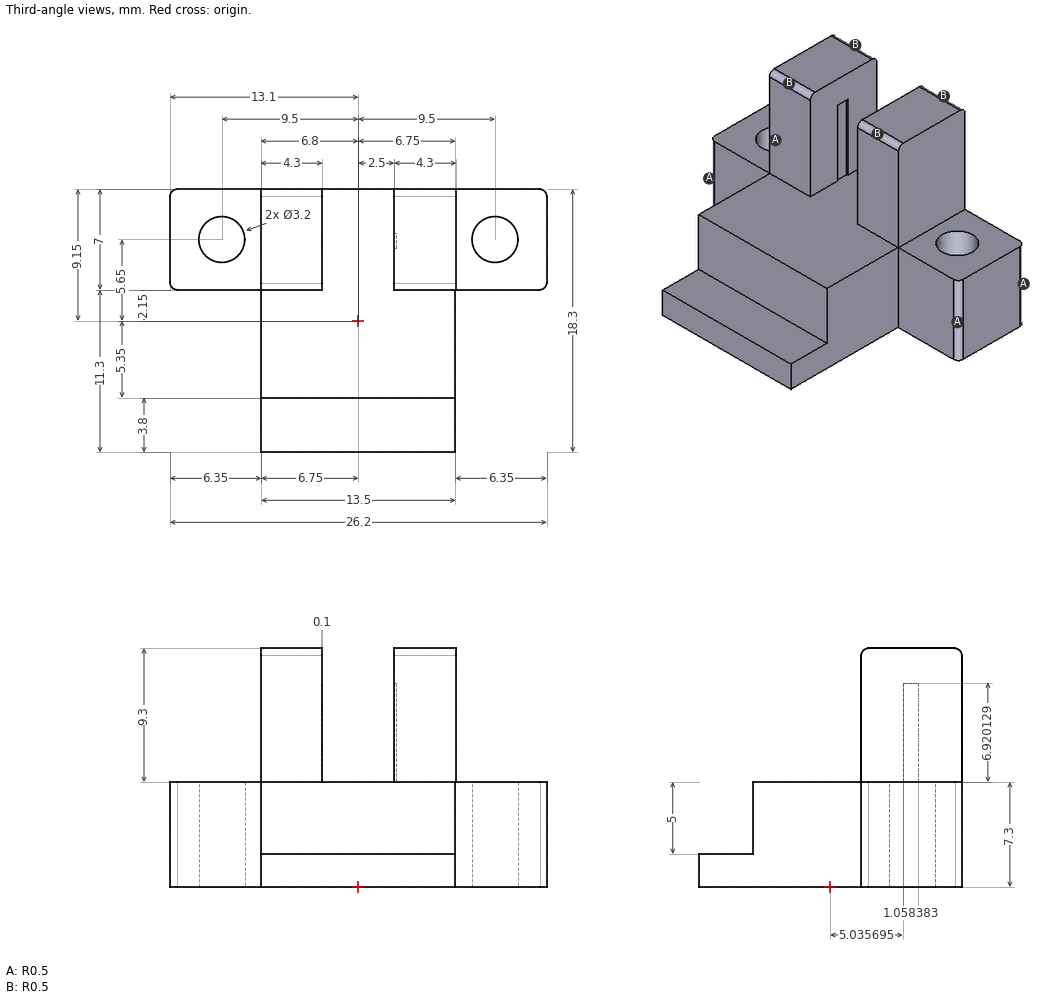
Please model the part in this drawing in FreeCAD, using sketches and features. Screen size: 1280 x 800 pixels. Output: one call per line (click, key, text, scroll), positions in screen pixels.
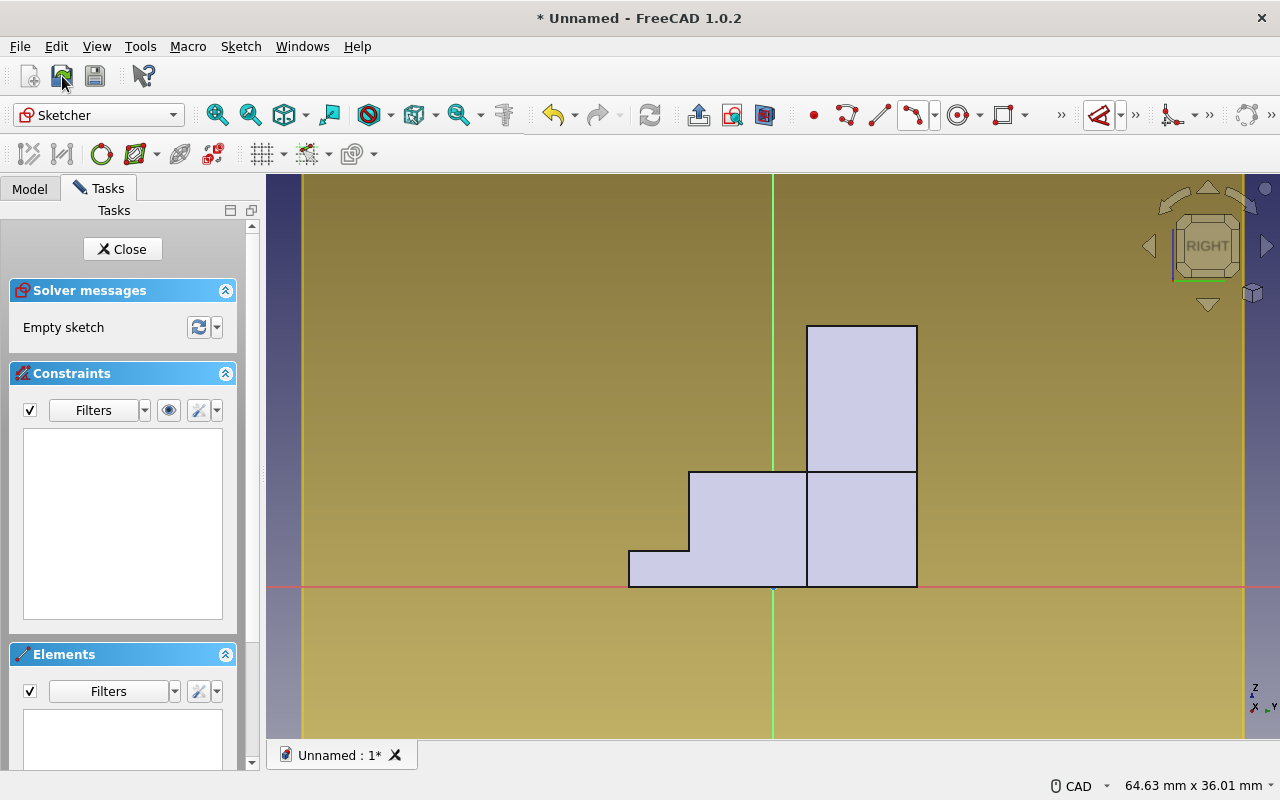
key(q)
key(s)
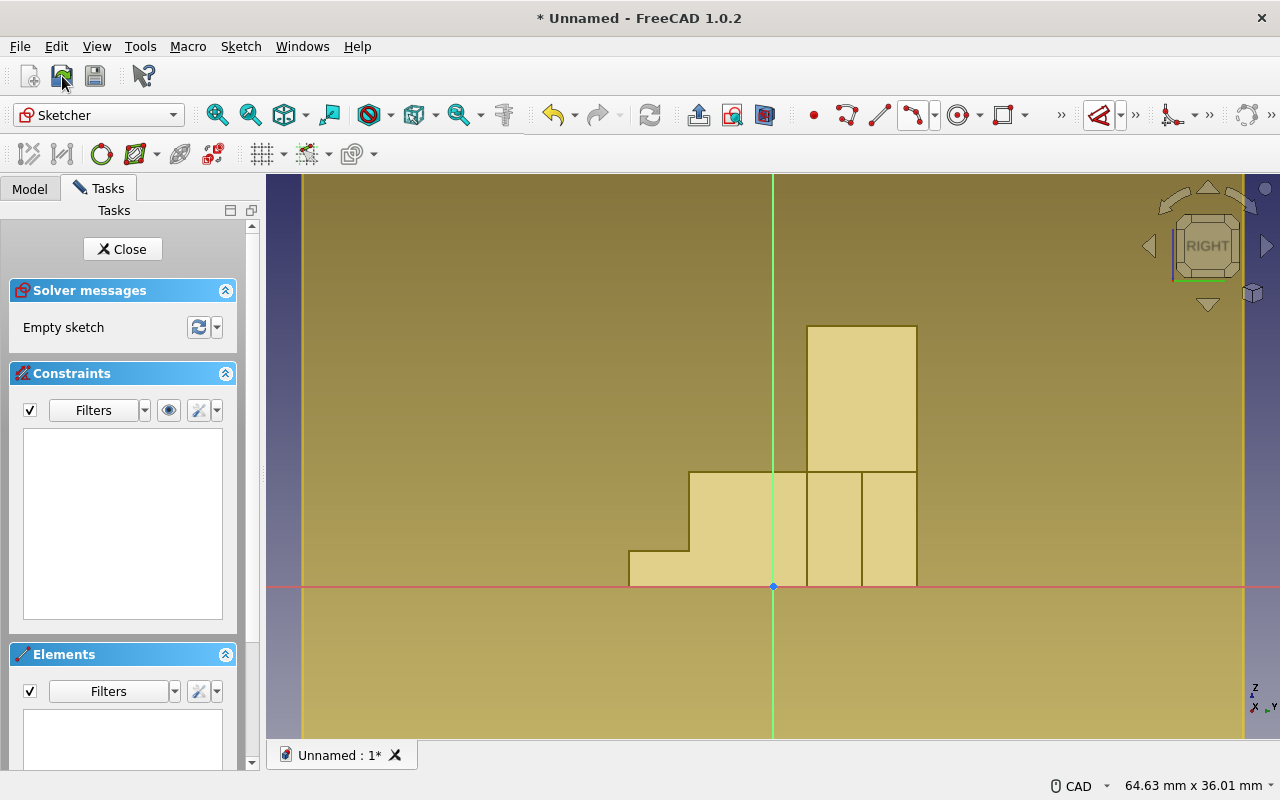
scroll(1057, 513, up, 2)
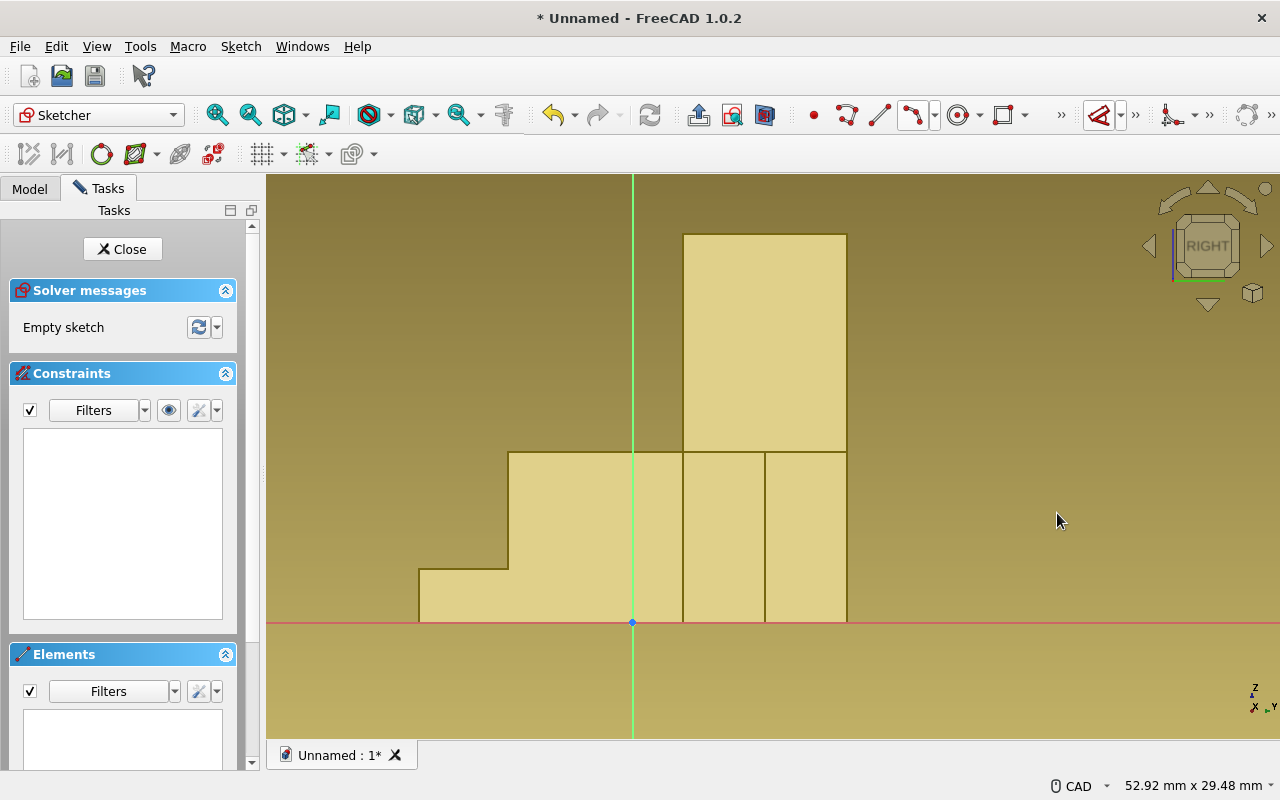
key(g)
key(r)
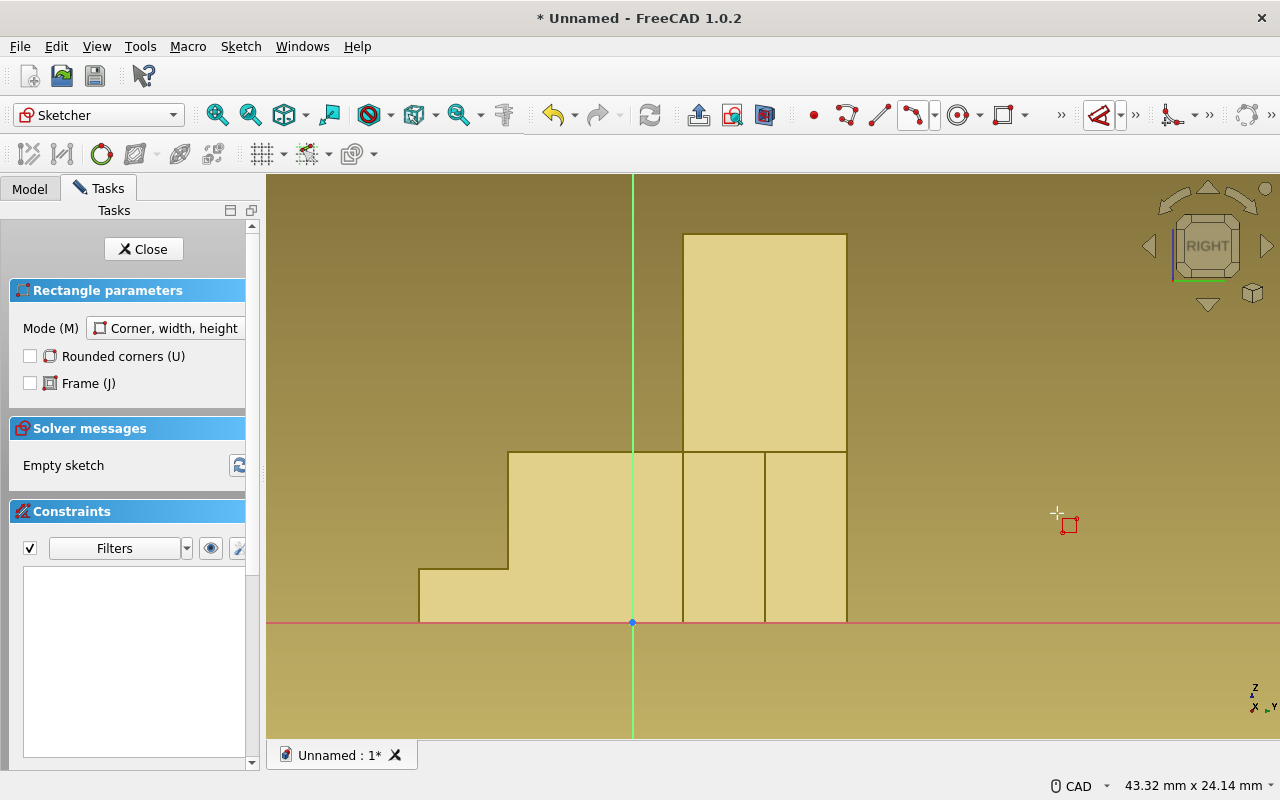
click(751, 290)
click(776, 452)
key(Escape)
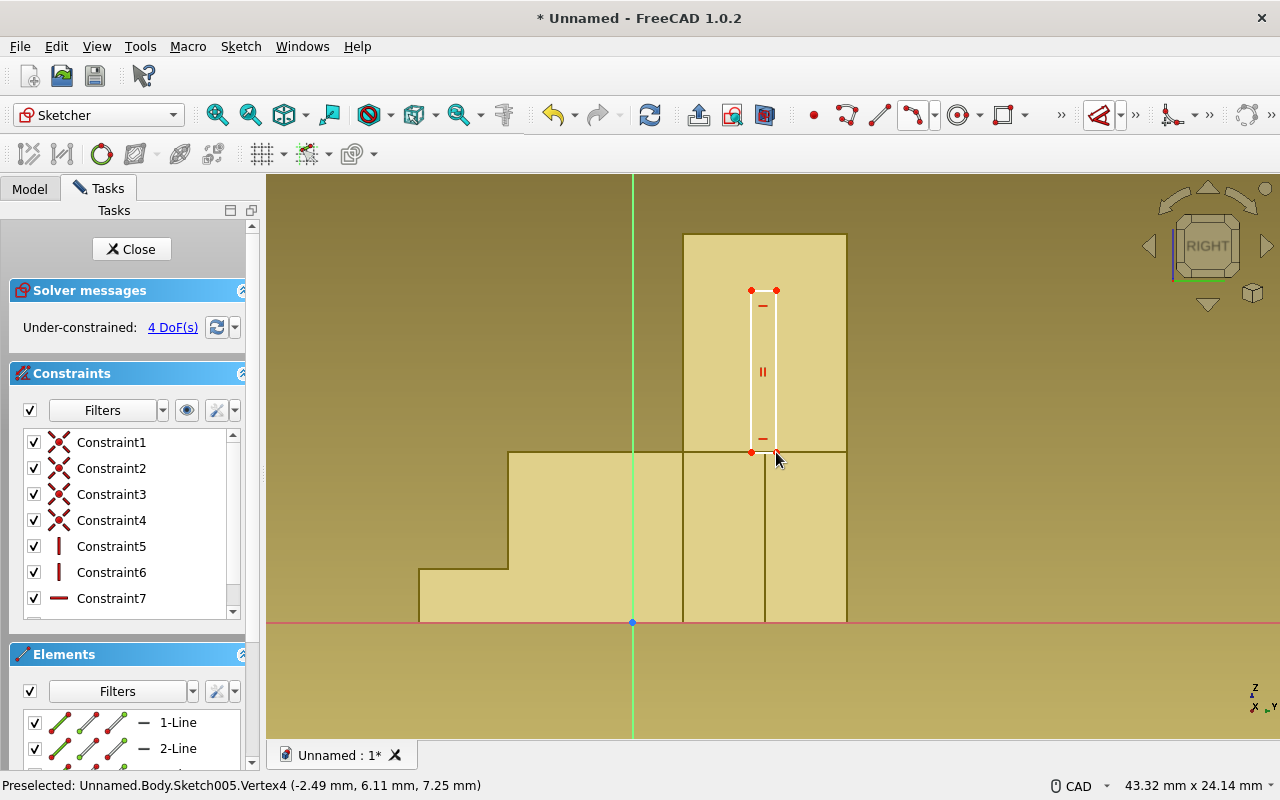
click(751, 453)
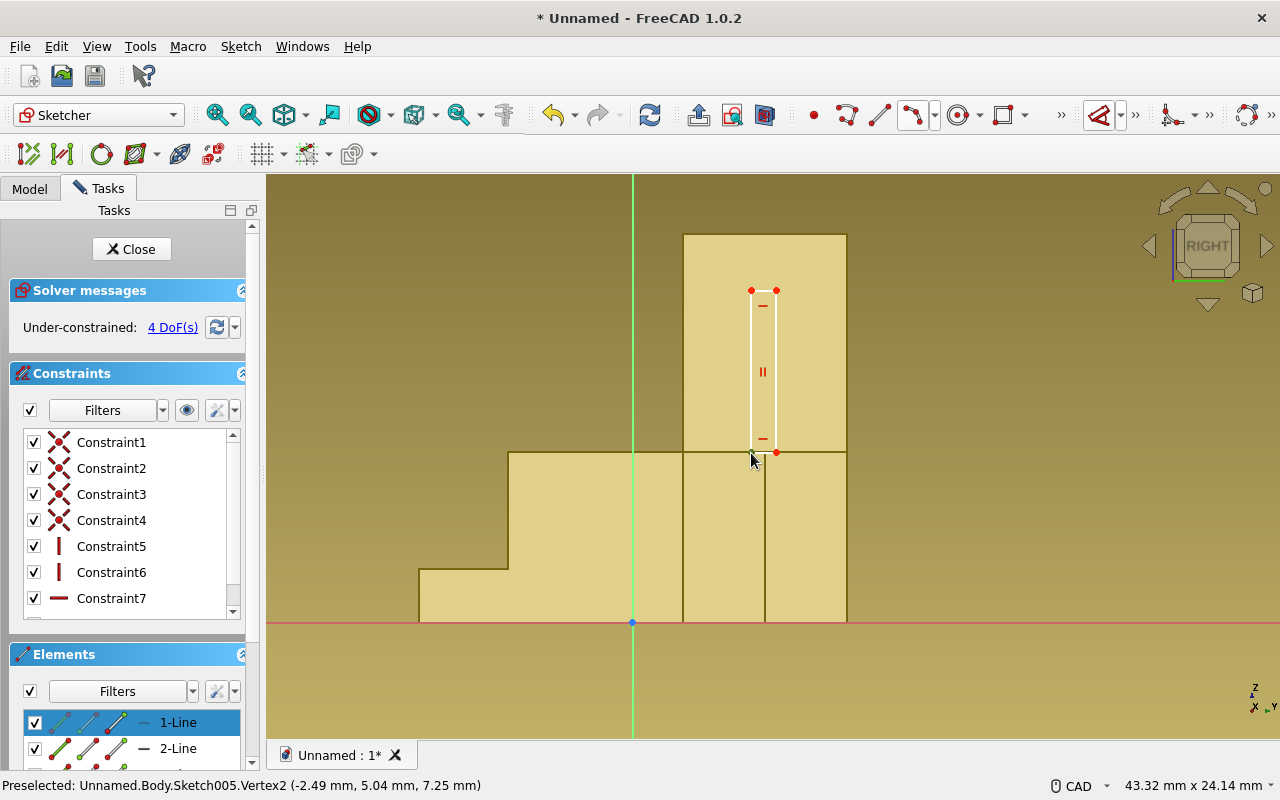
key(i)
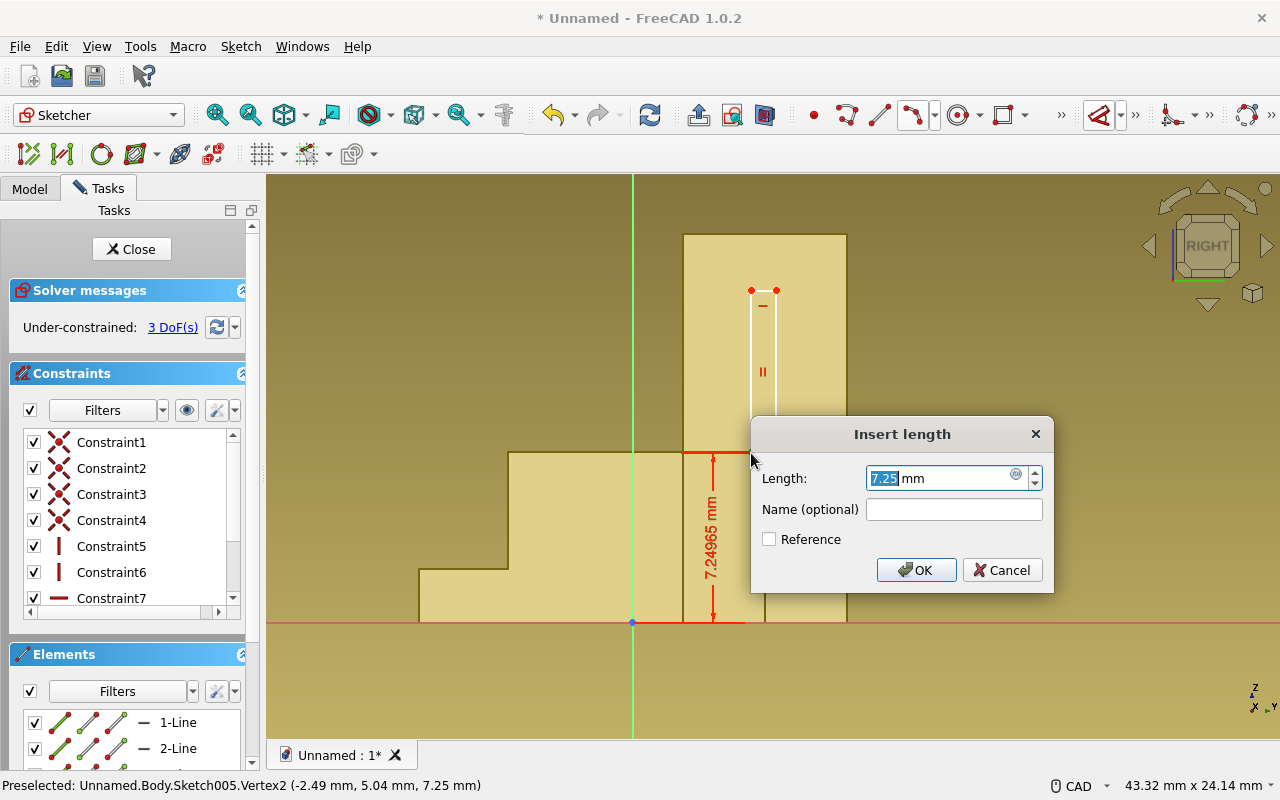
text(7.3)
key(Return)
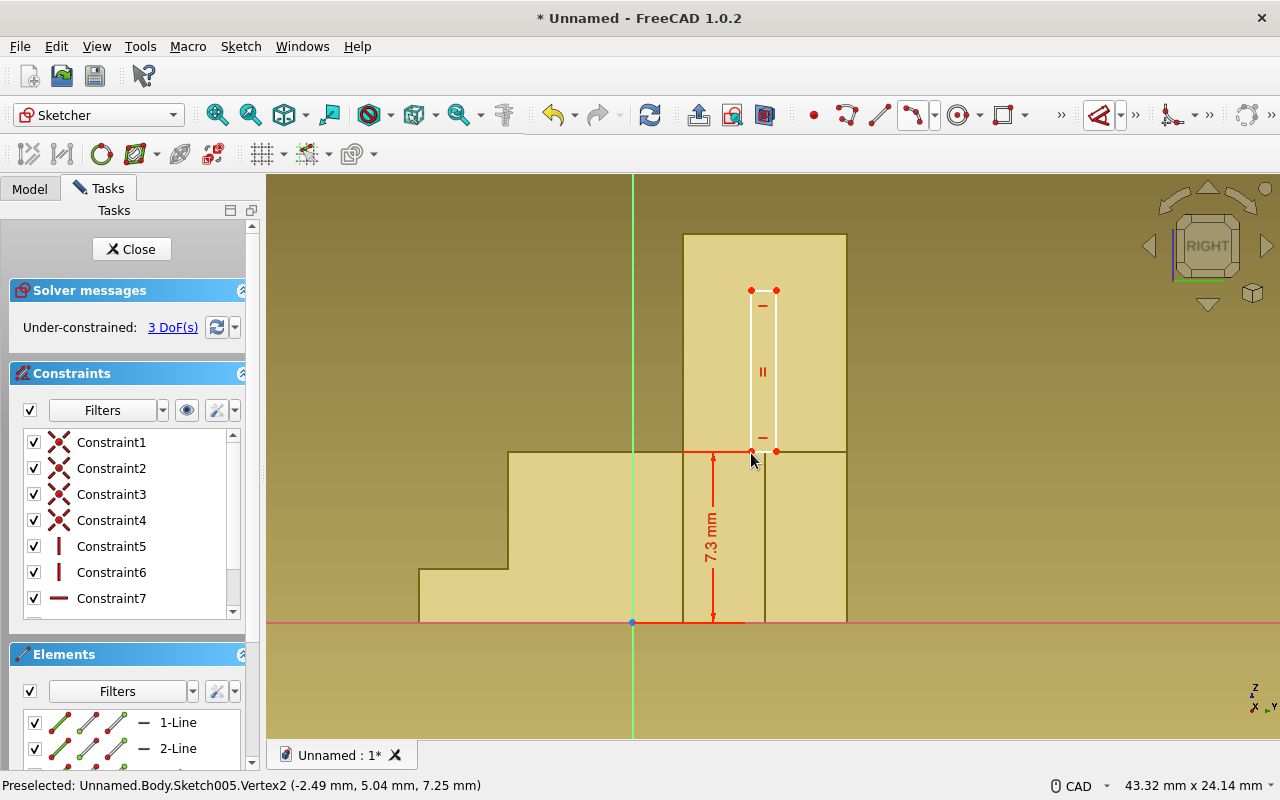
click(751, 339)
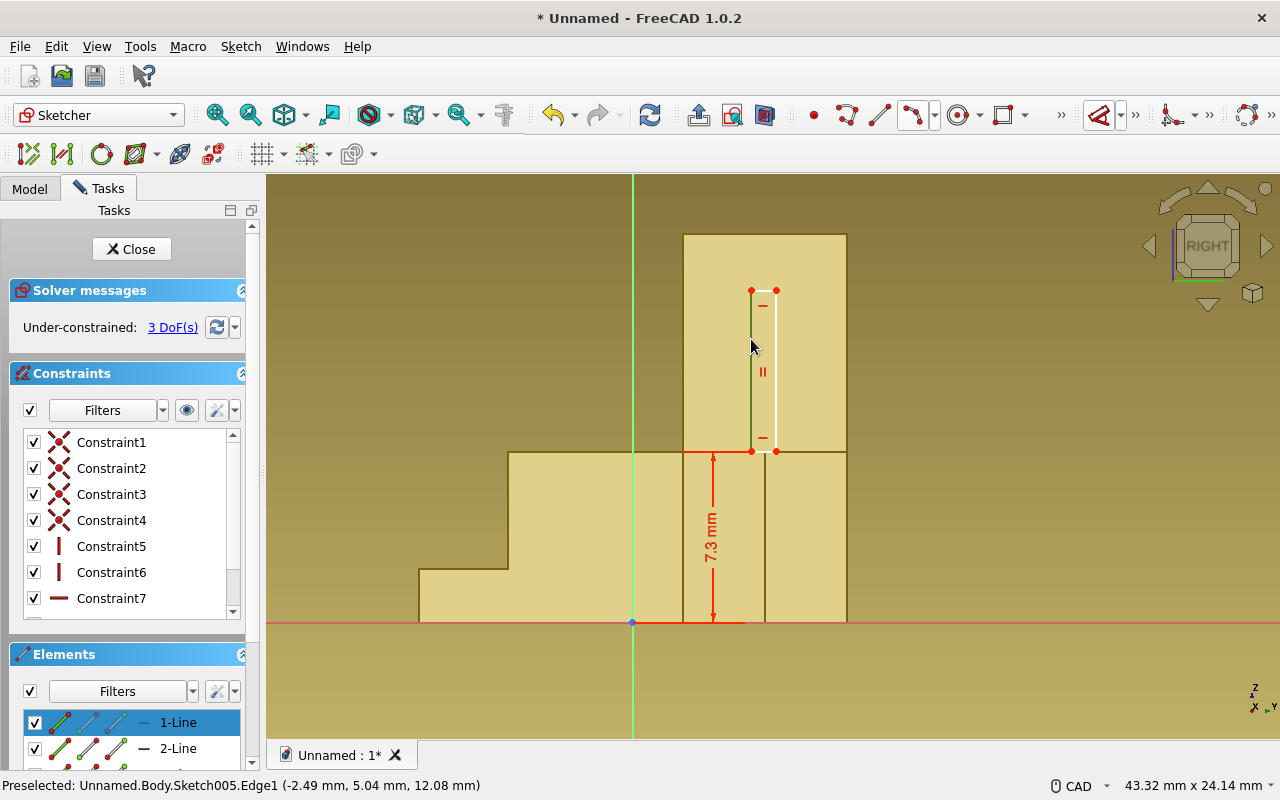
key(i)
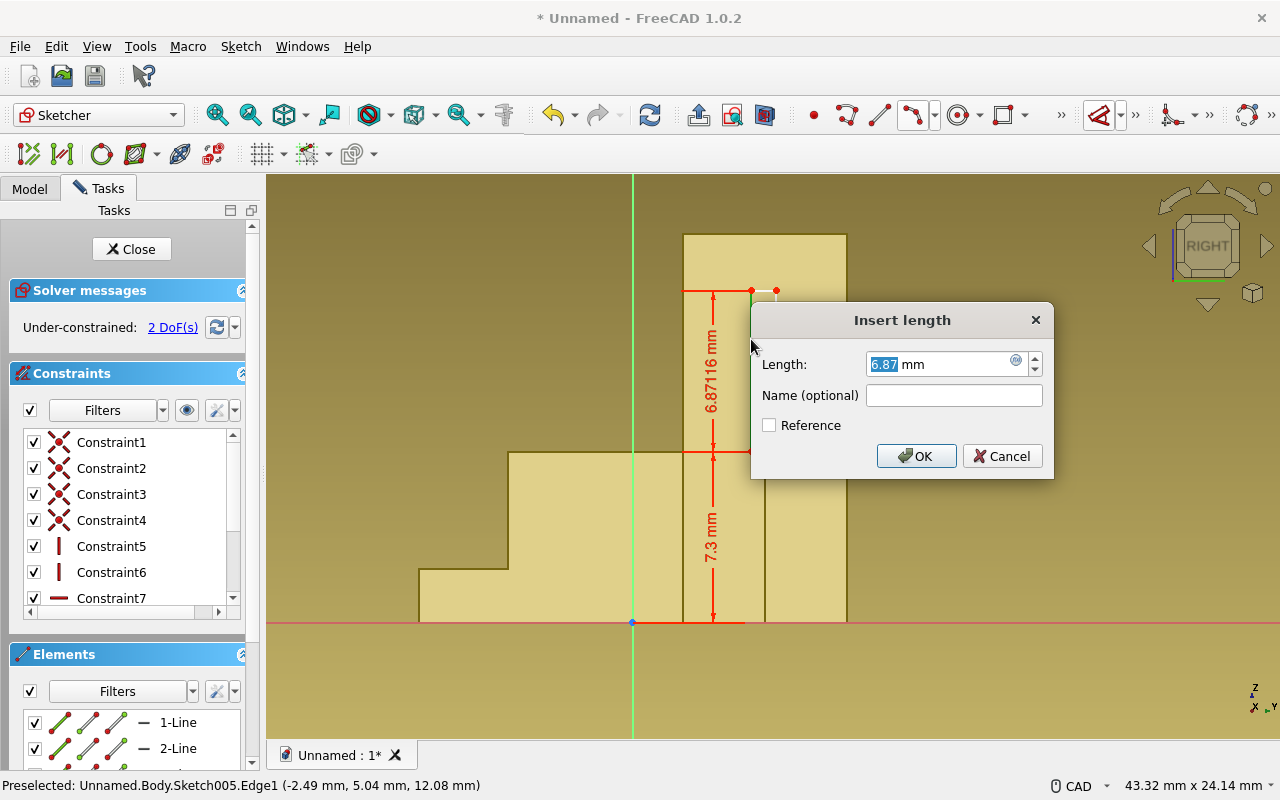
text(6.920129)
key(Return)